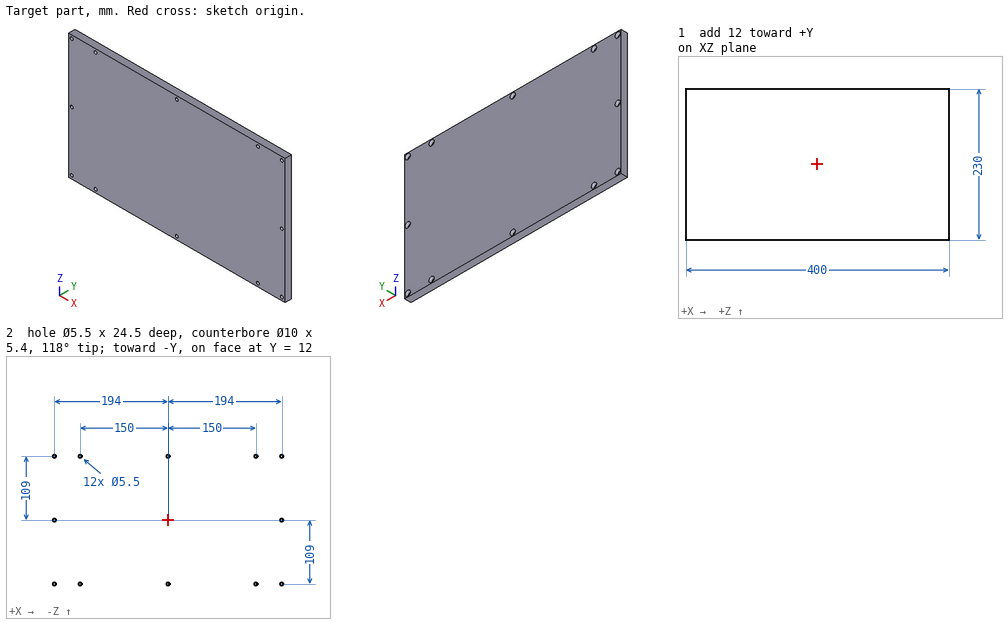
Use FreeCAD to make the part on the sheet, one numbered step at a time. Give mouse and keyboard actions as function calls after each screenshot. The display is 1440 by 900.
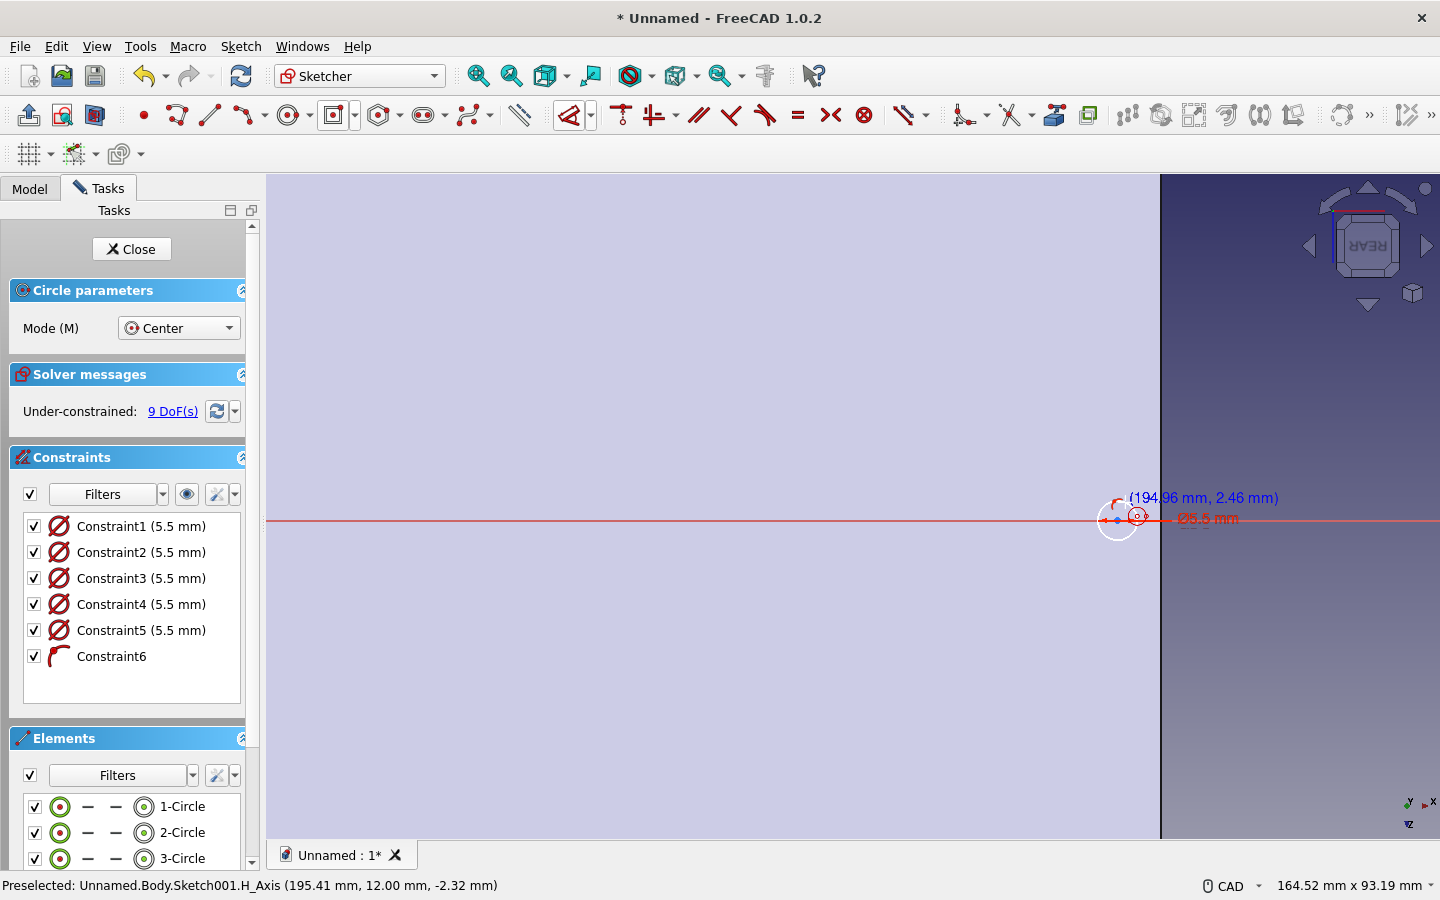
scroll(1128, 502, down, 7)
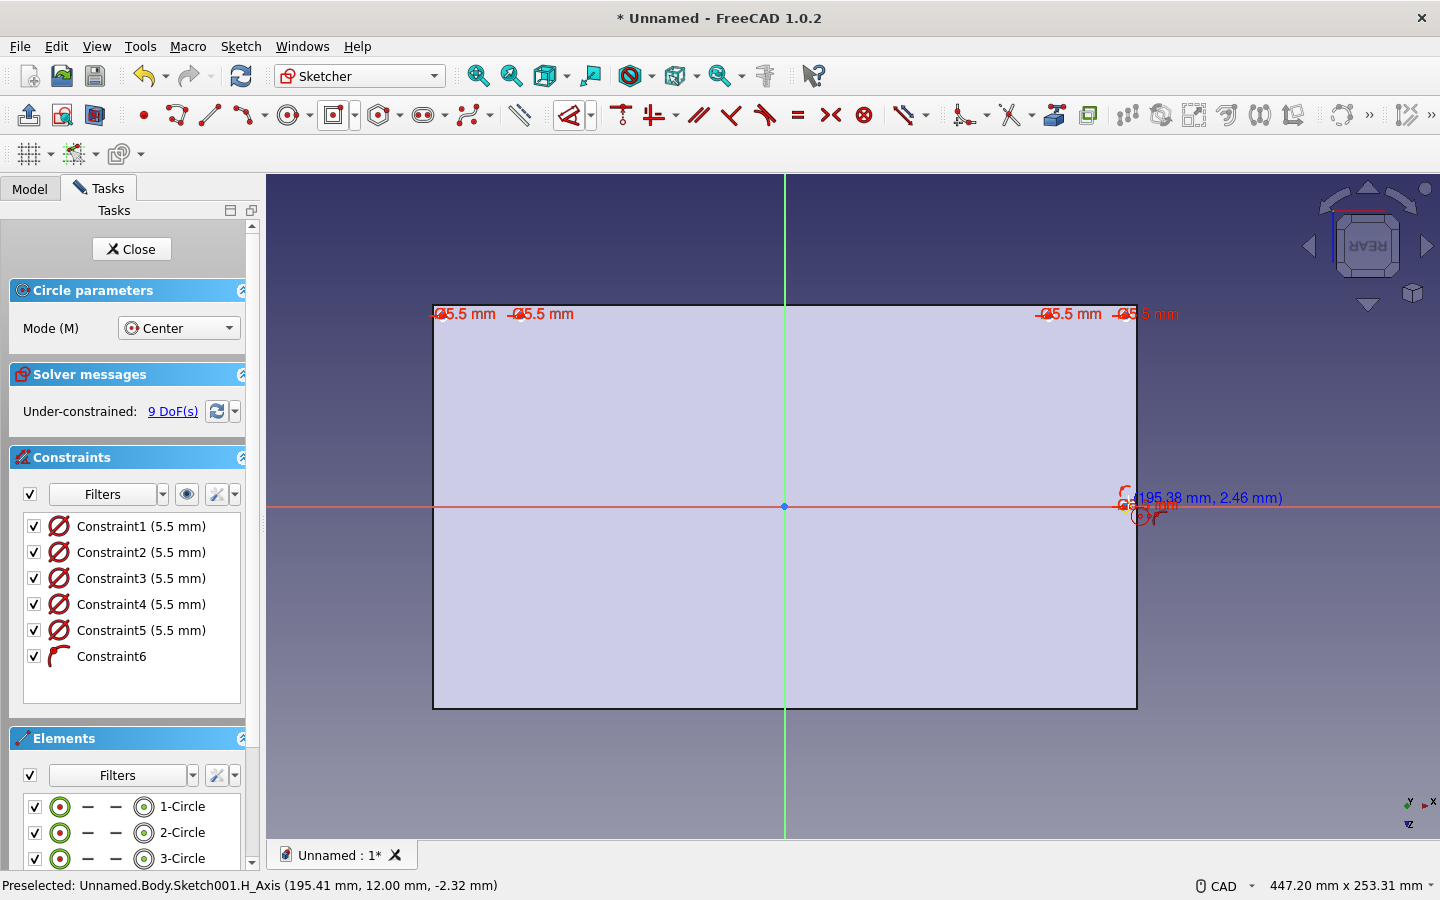
scroll(1126, 699, up, 8)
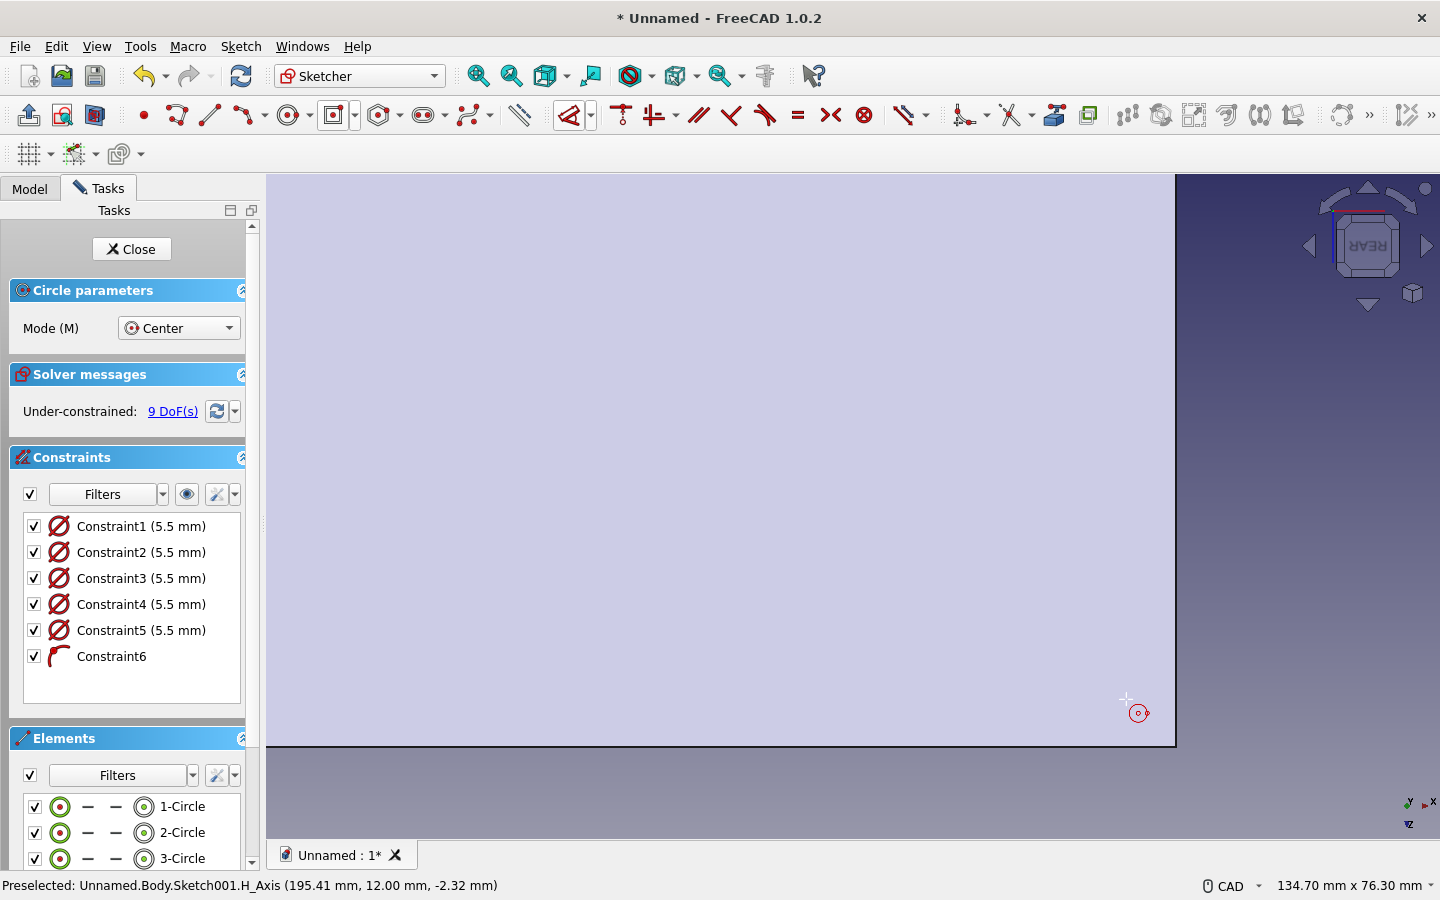
scroll(1126, 699, down, 8)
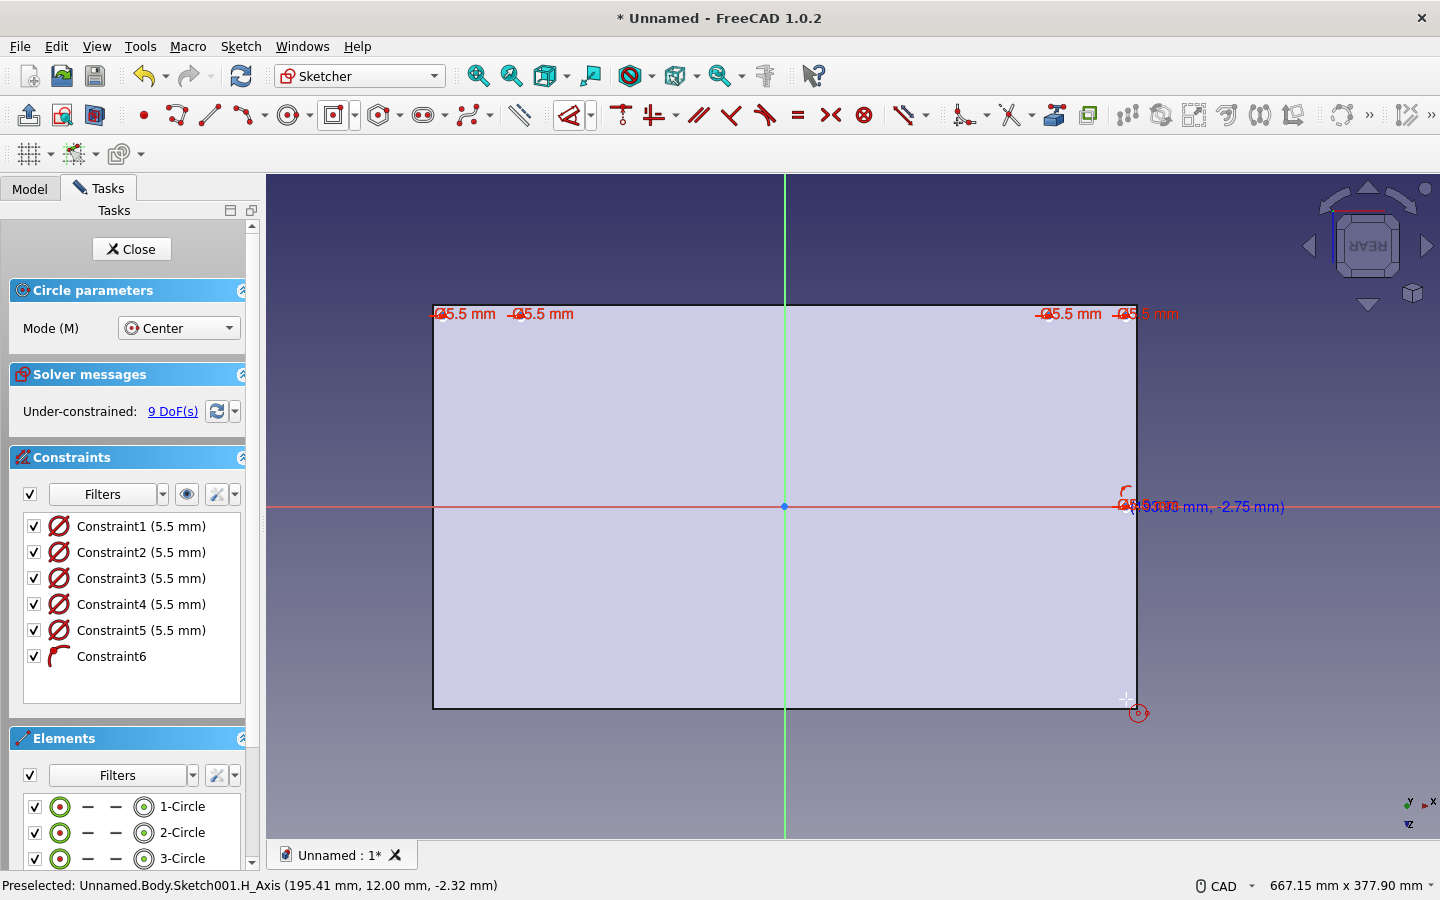
click(1126, 699)
move(1130, 695)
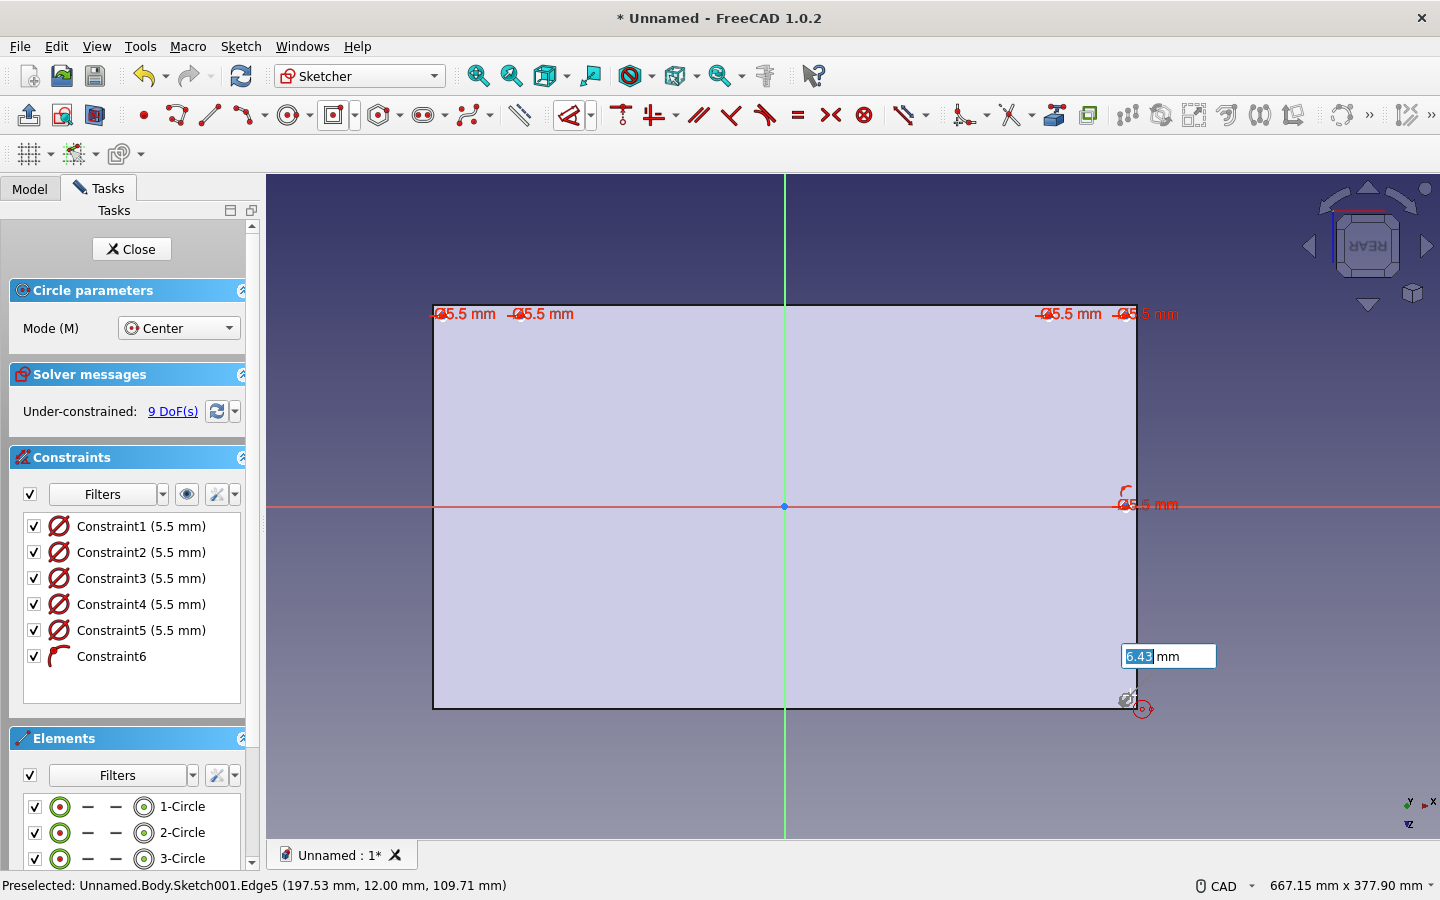
text(5.5)
key(Return)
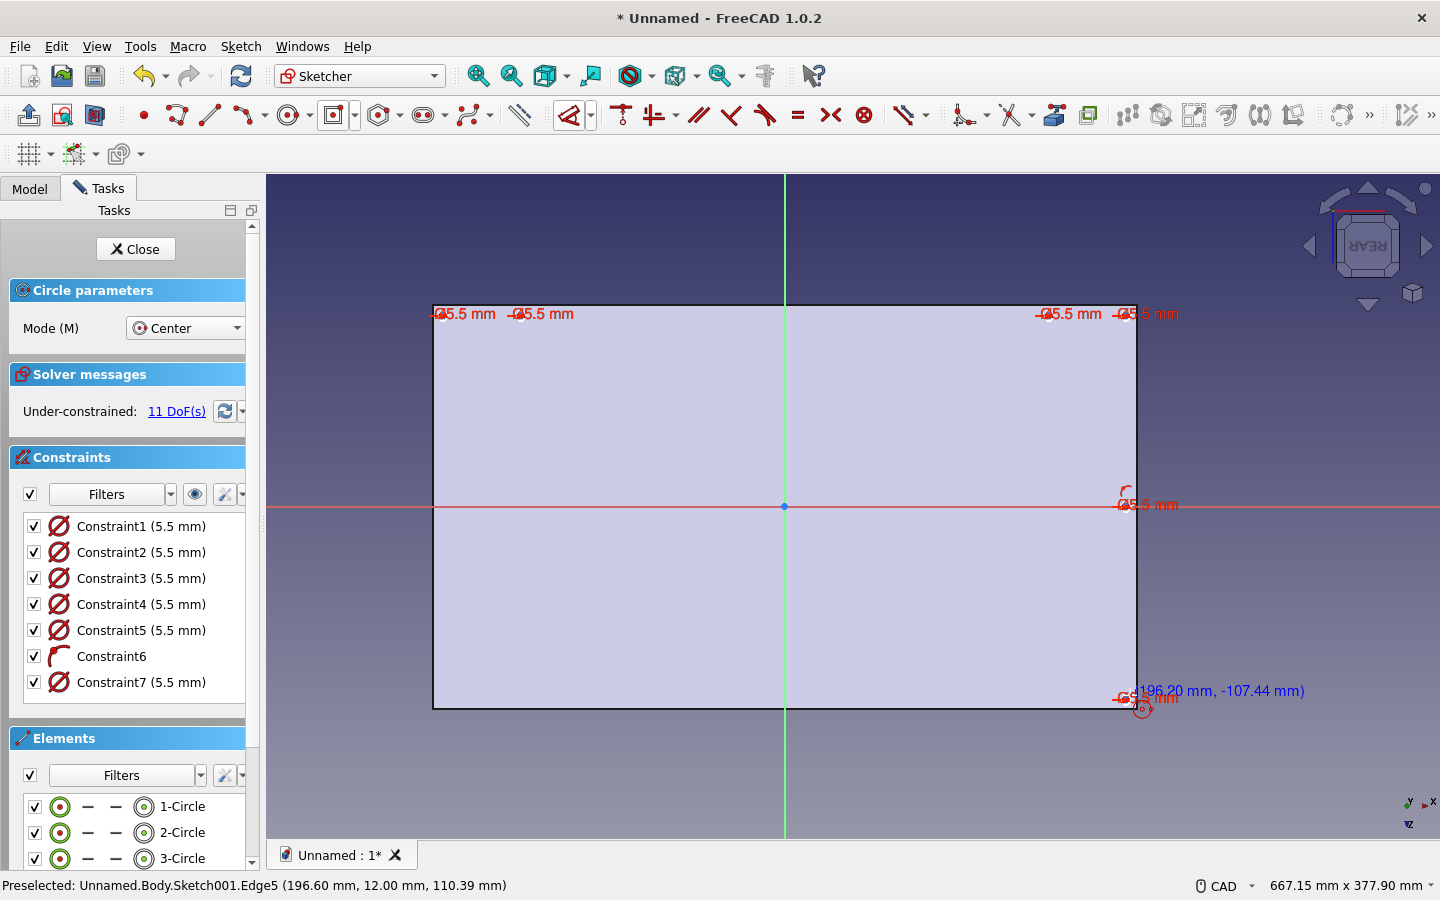
scroll(1049, 699, up, 8)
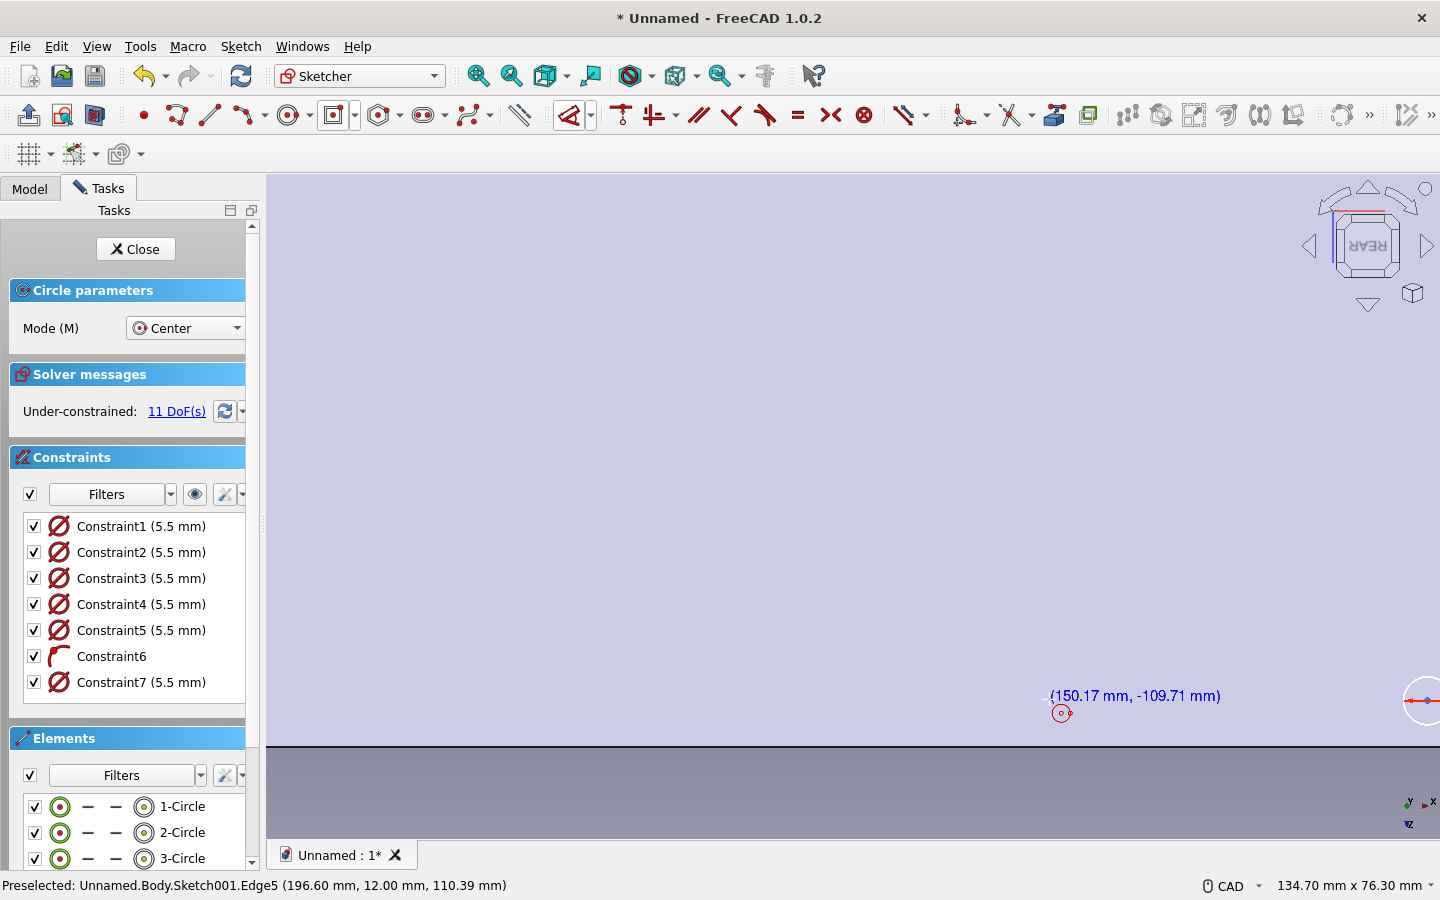
scroll(1049, 699, down, 8)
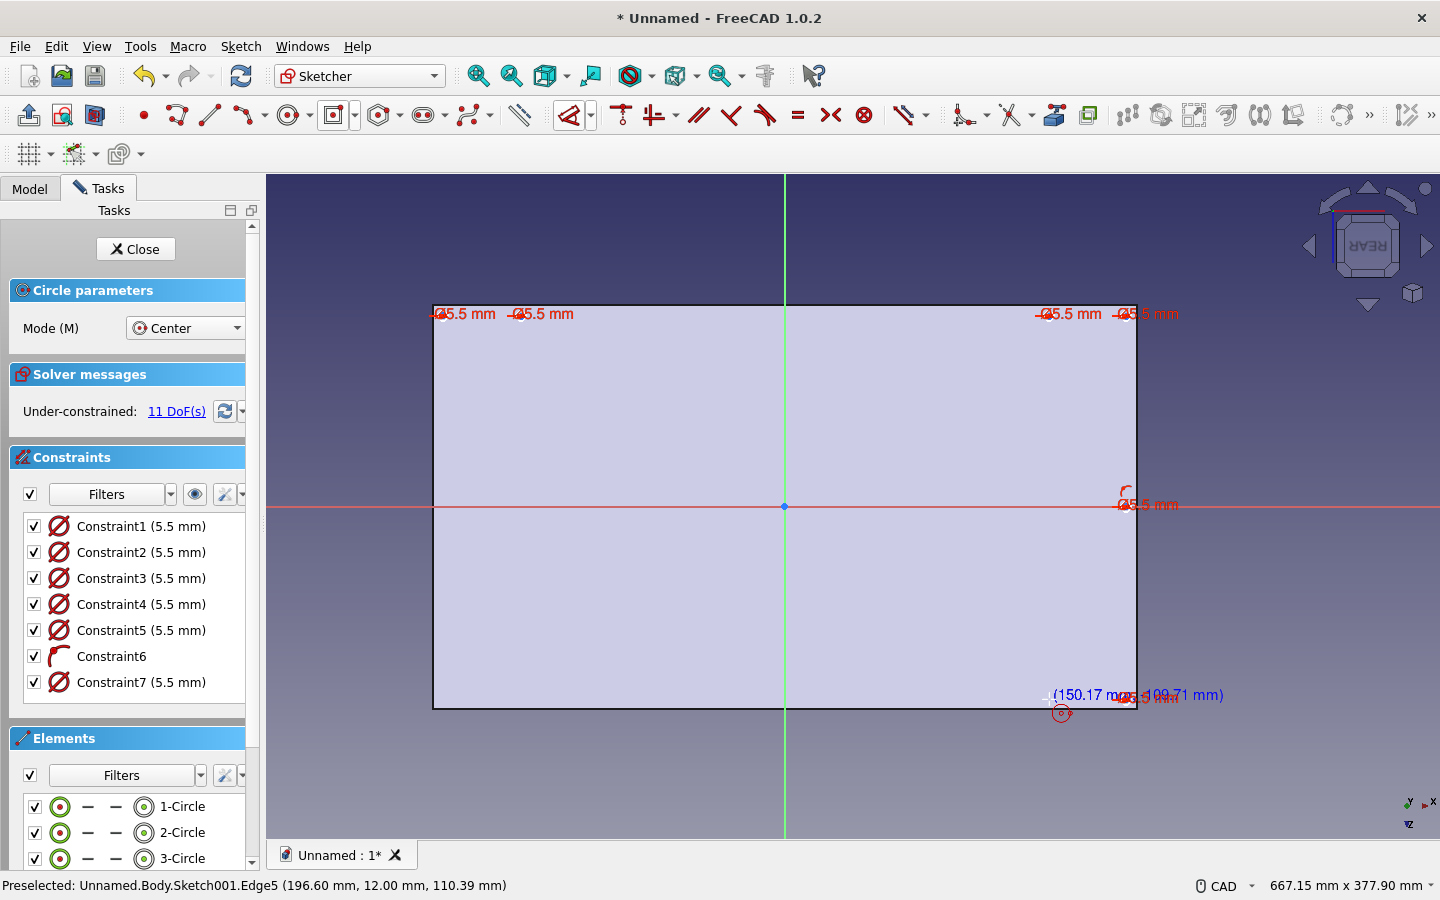
click(1049, 699)
move(1052, 695)